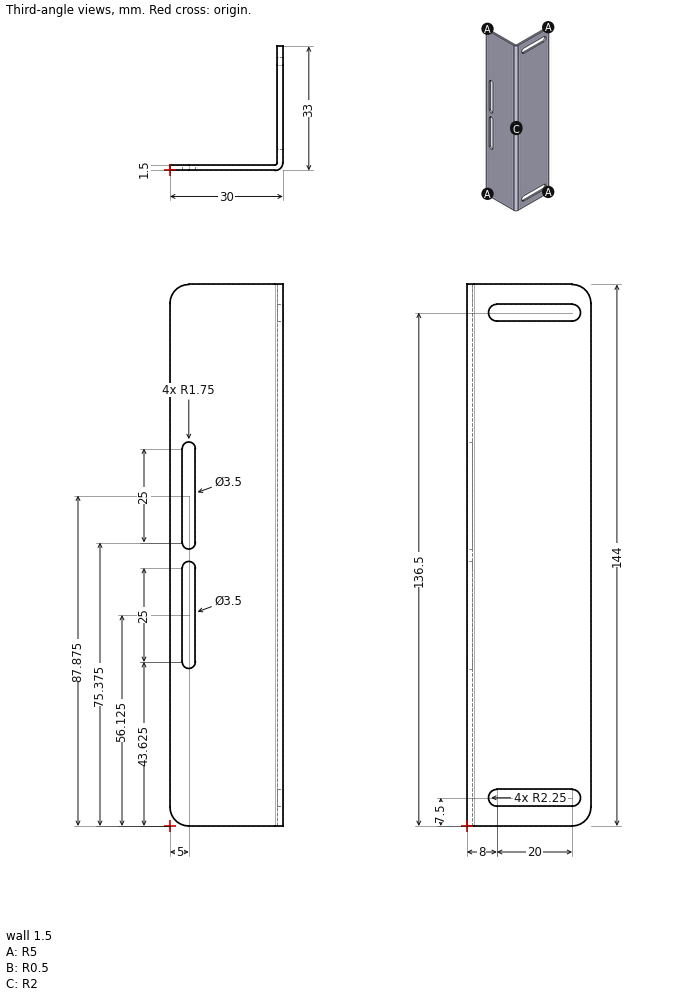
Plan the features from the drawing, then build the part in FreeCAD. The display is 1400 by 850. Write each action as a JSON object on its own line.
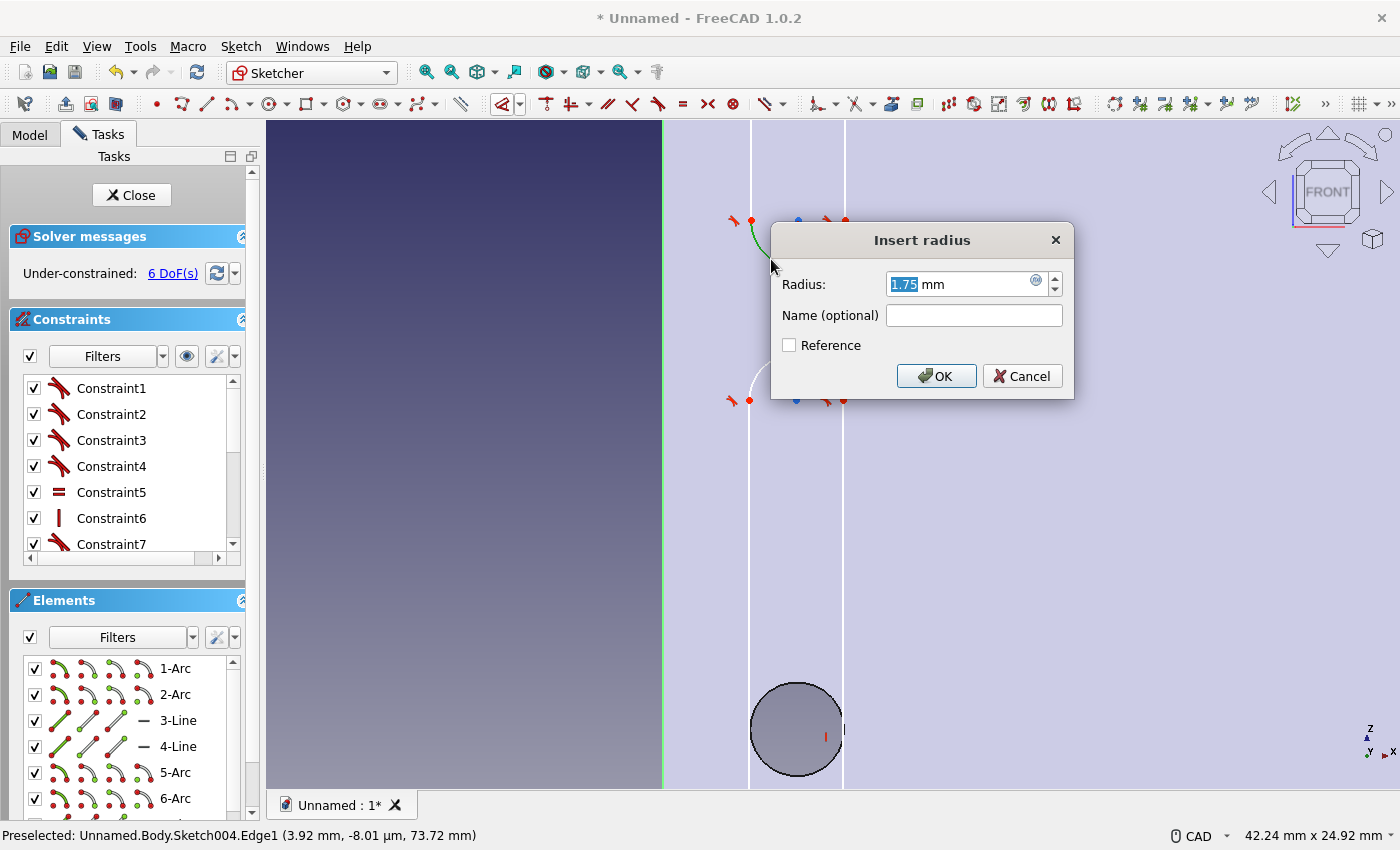
{"action": "type", "text": "1.75"}
{"action": "key", "text": "Return"}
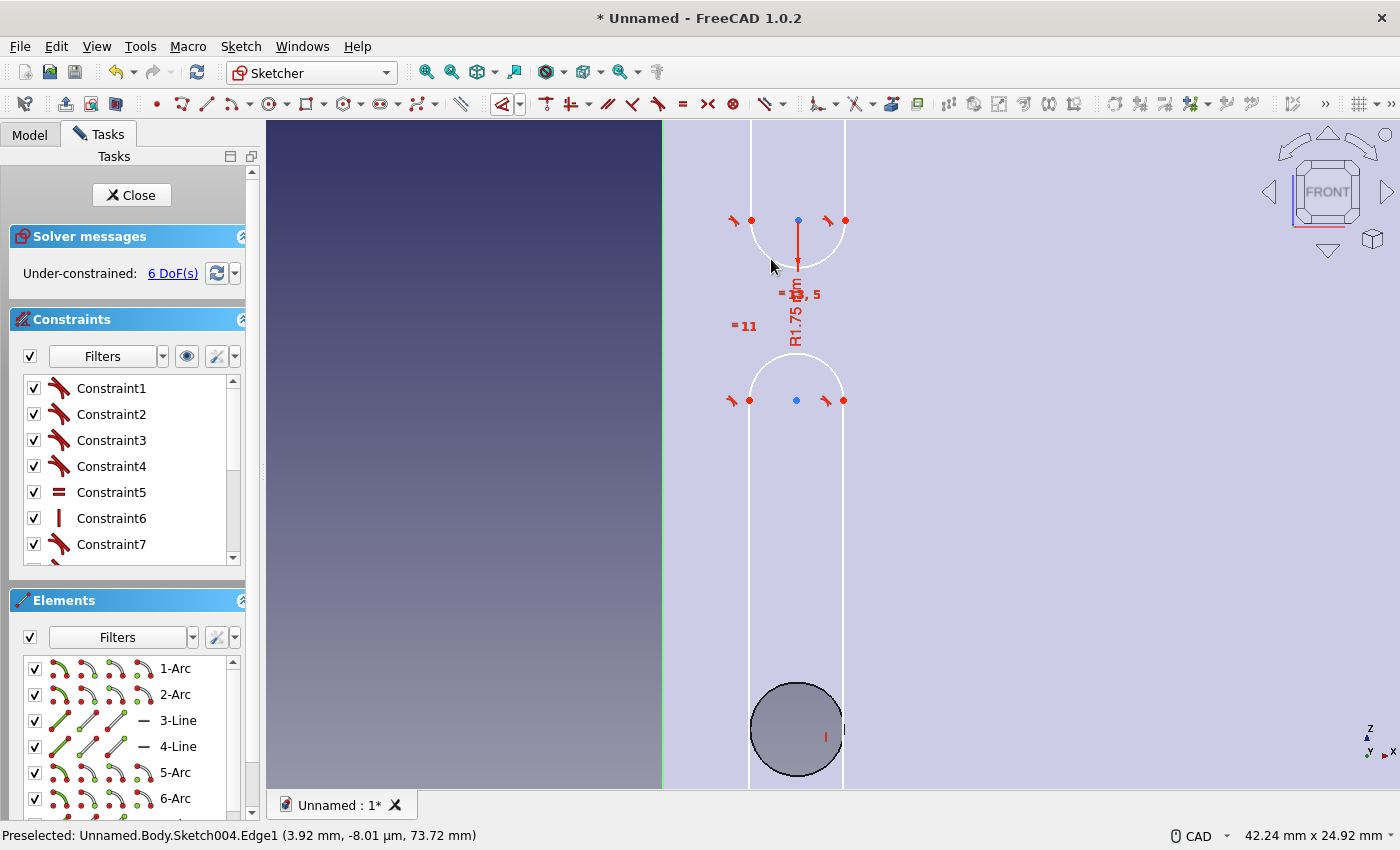
{"action": "scroll", "coordinate": [767, 373], "scroll_direction": "down", "scroll_amount": 9}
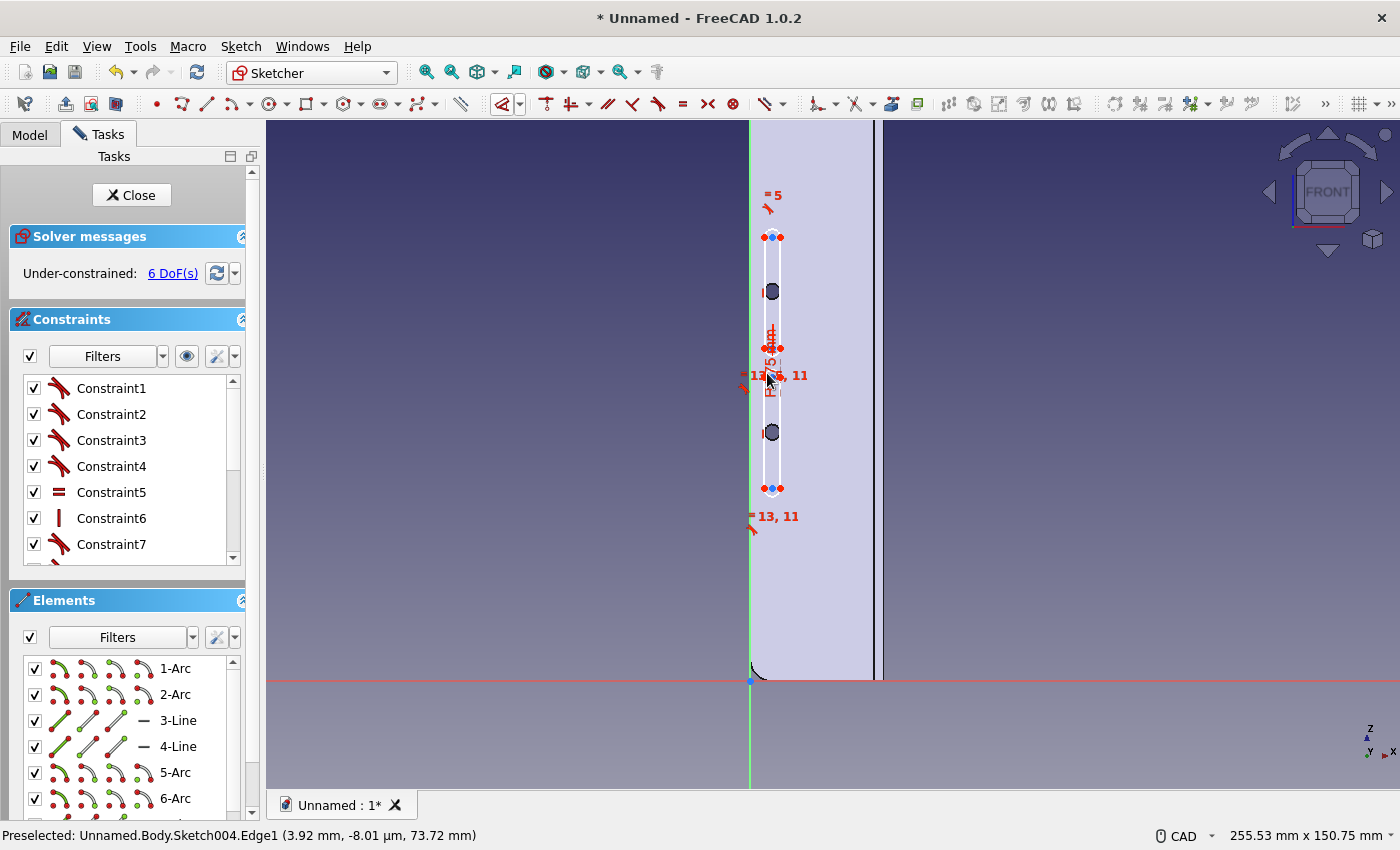
{"action": "left_click", "coordinate": [765, 315]}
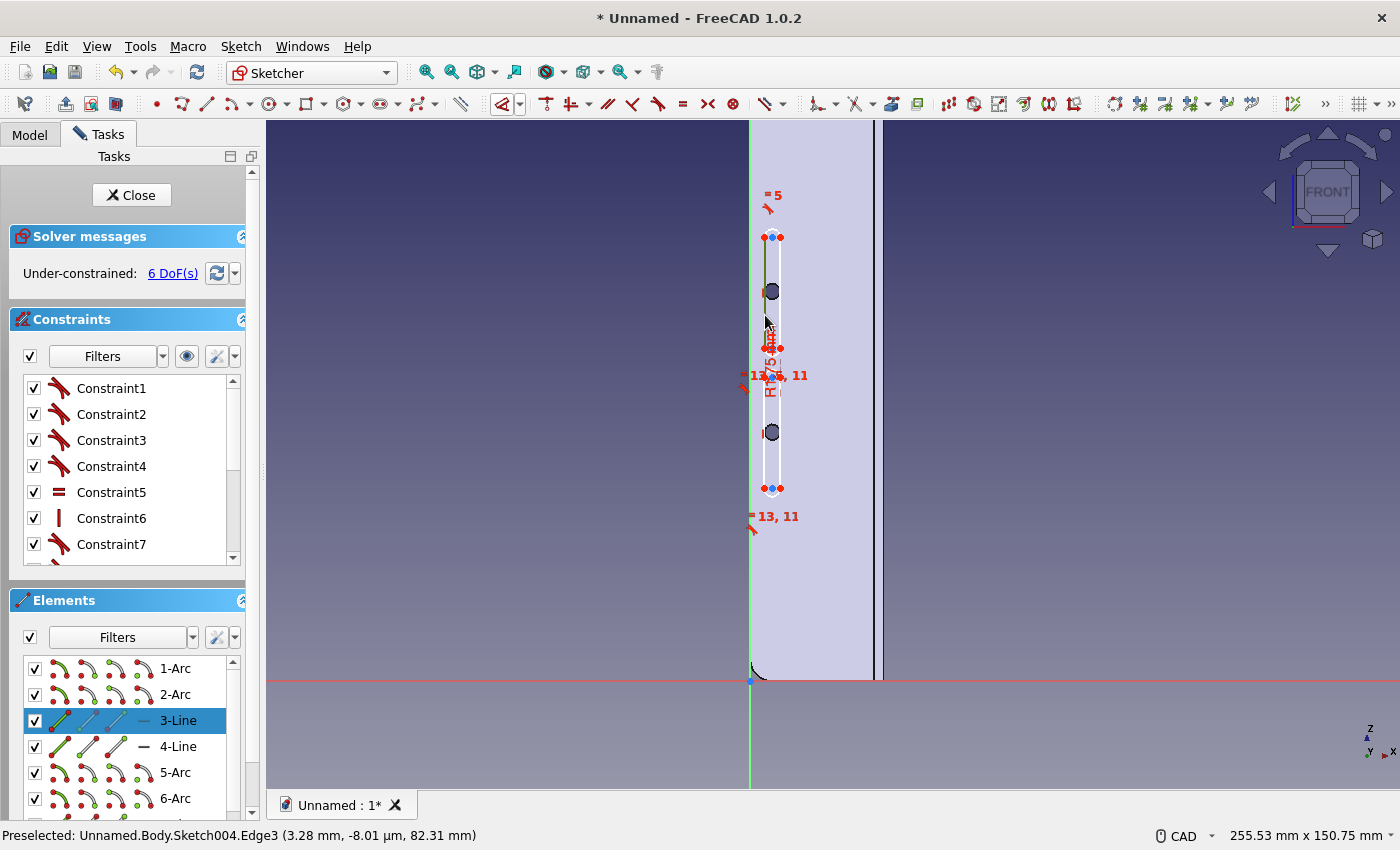
{"action": "key", "text": "i"}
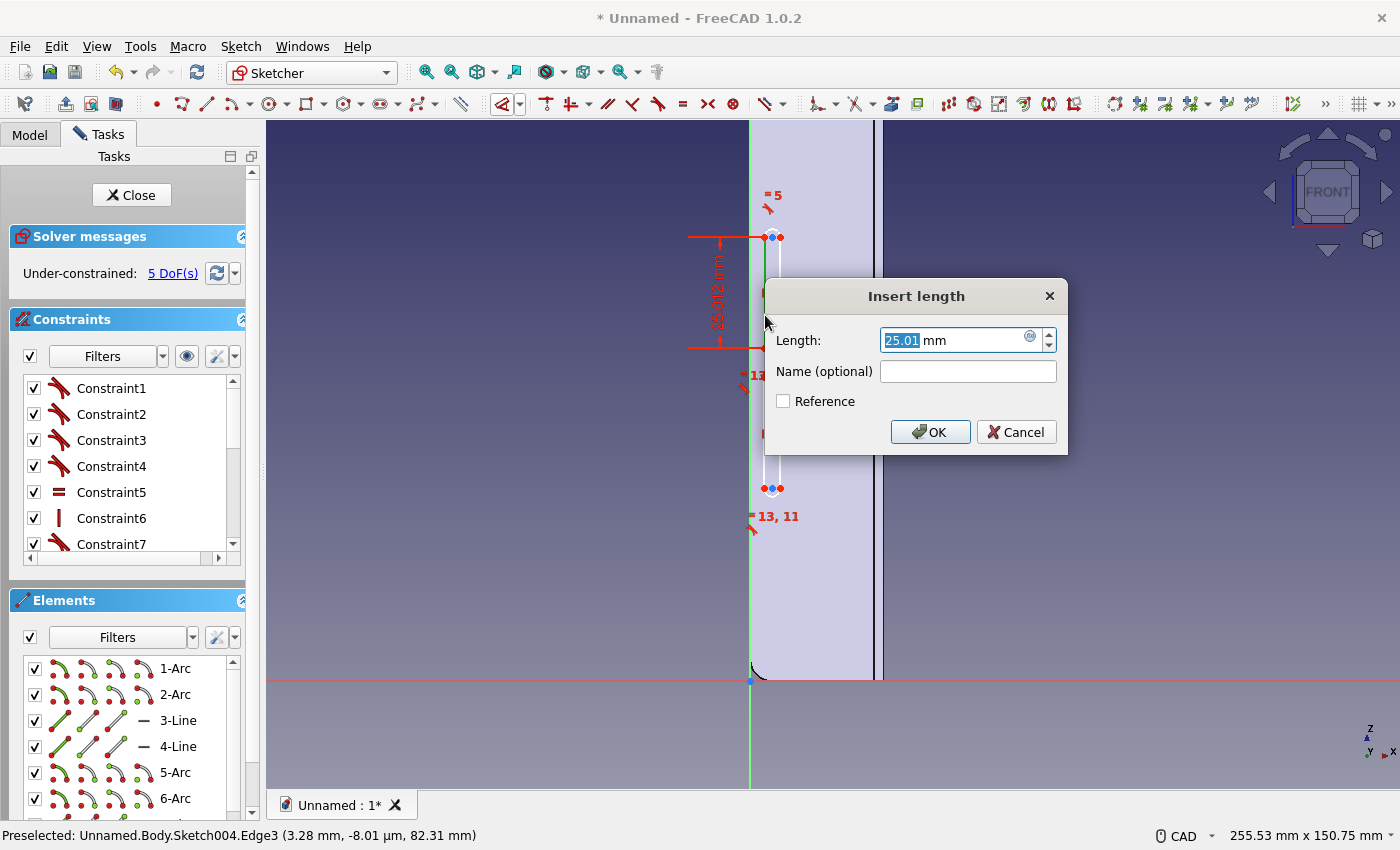
{"action": "type", "text": "25"}
{"action": "key", "text": "Return"}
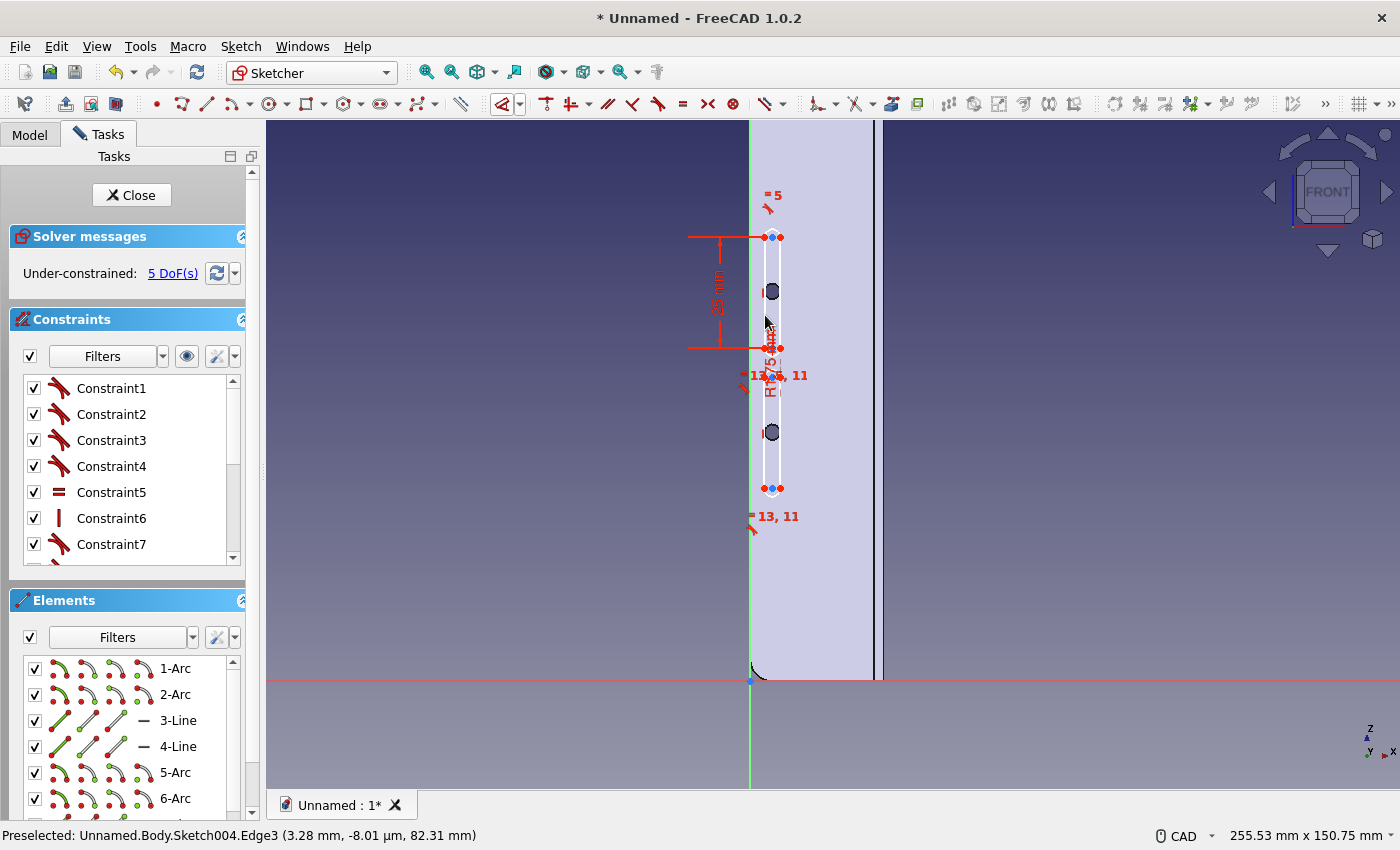
{"action": "left_click", "coordinate": [764, 456]}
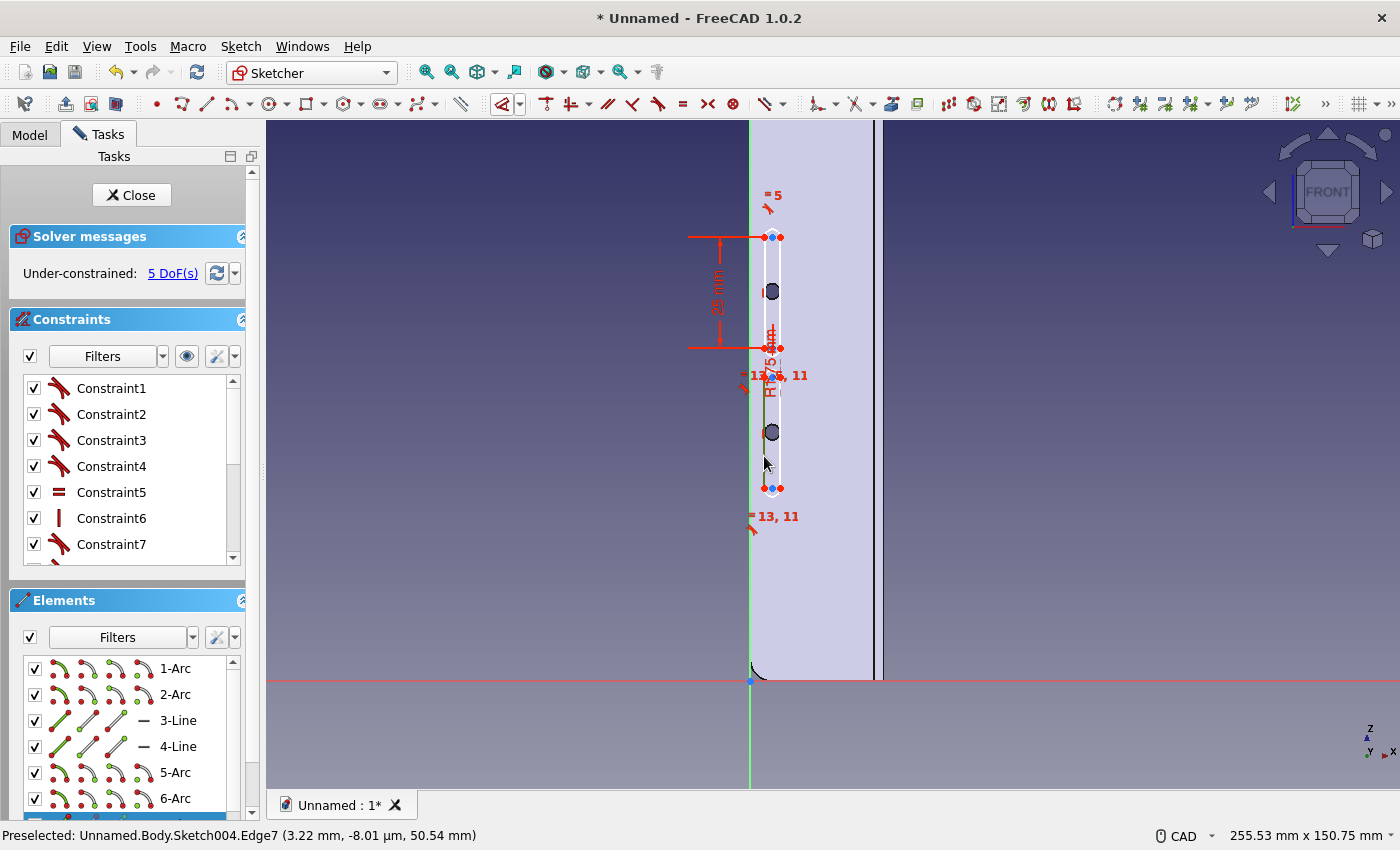
{"action": "left_click", "coordinate": [520, 104]}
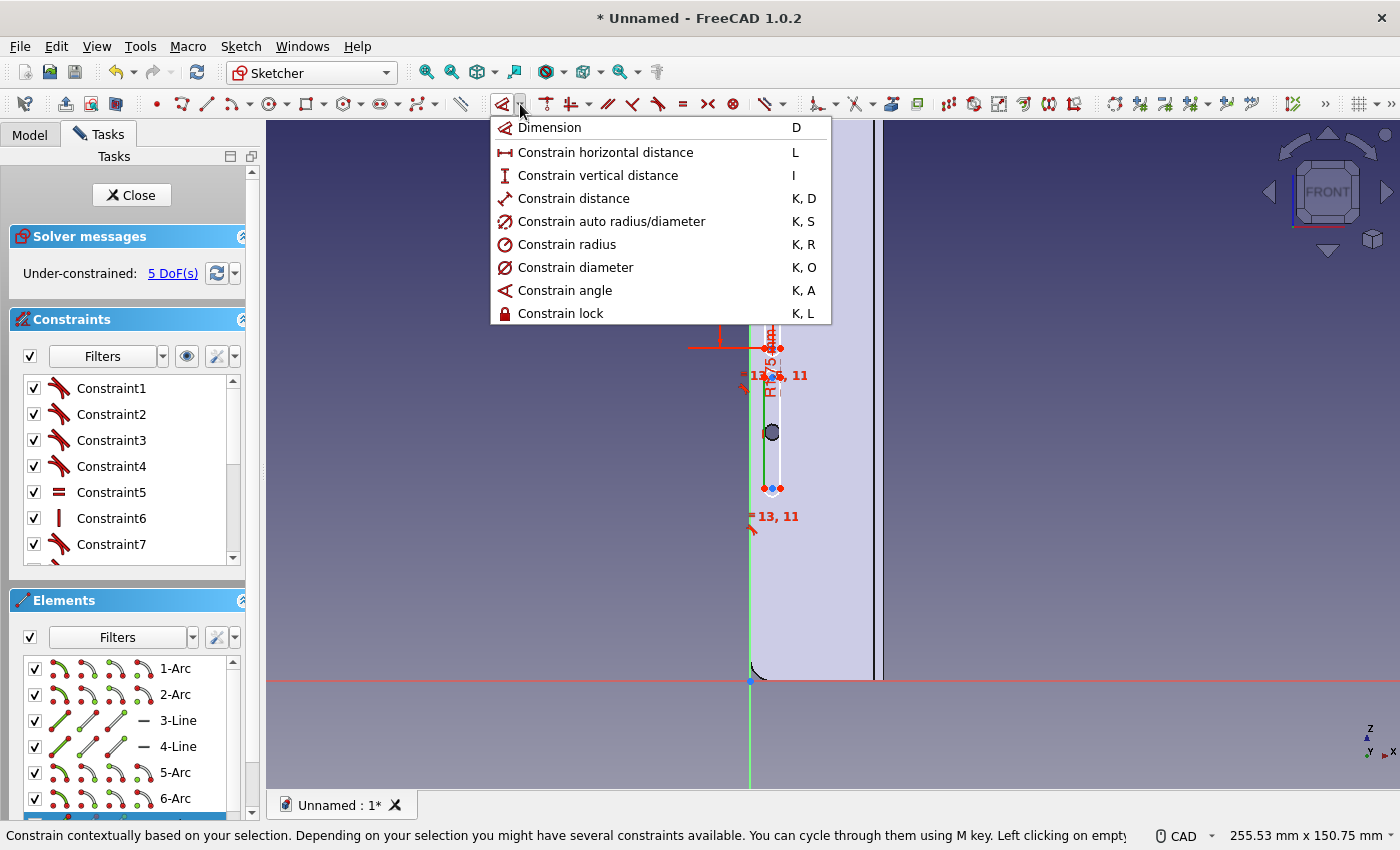
{"action": "left_click", "coordinate": [661, 176]}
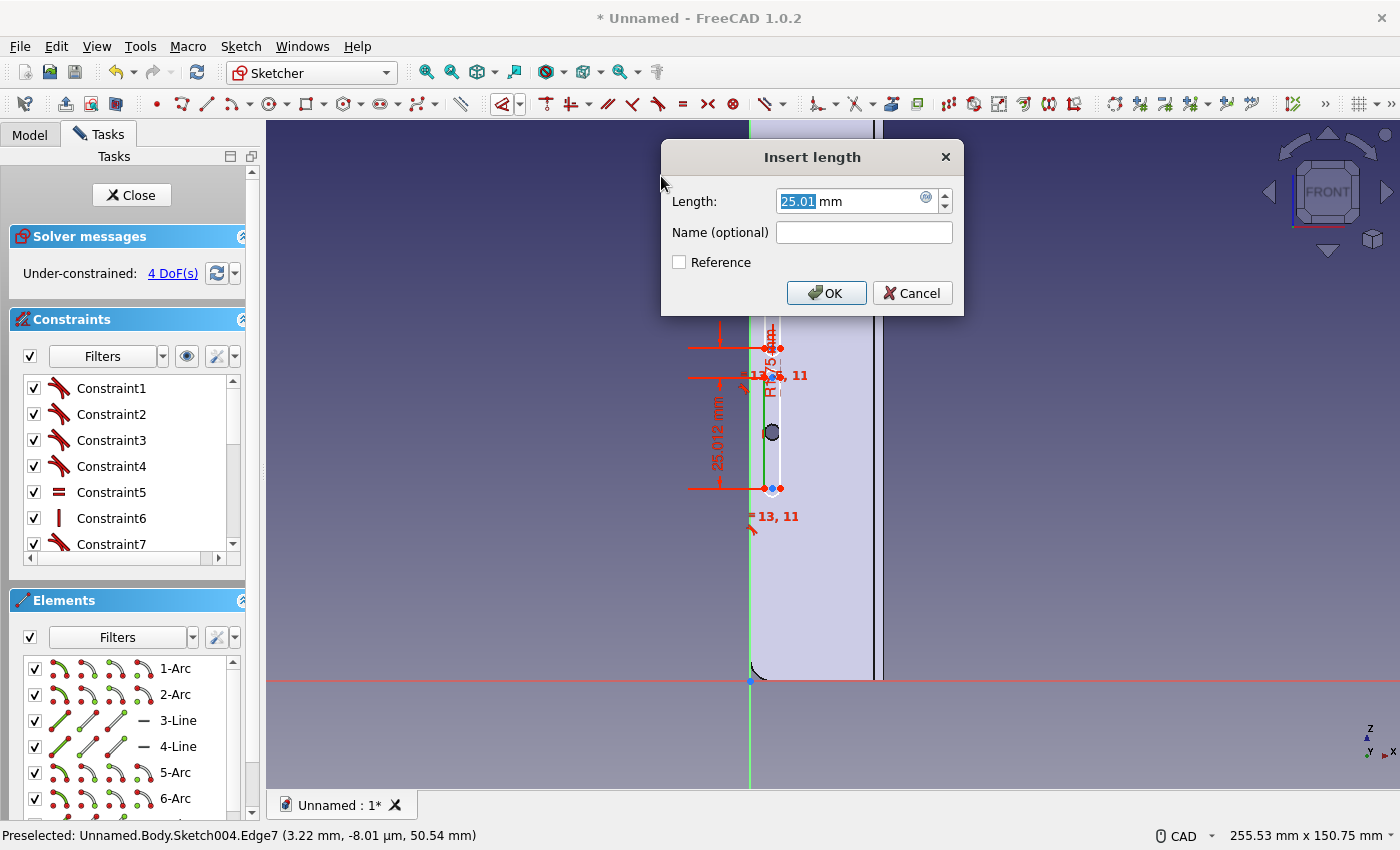
{"action": "type", "text": "25"}
{"action": "key", "text": "Return"}